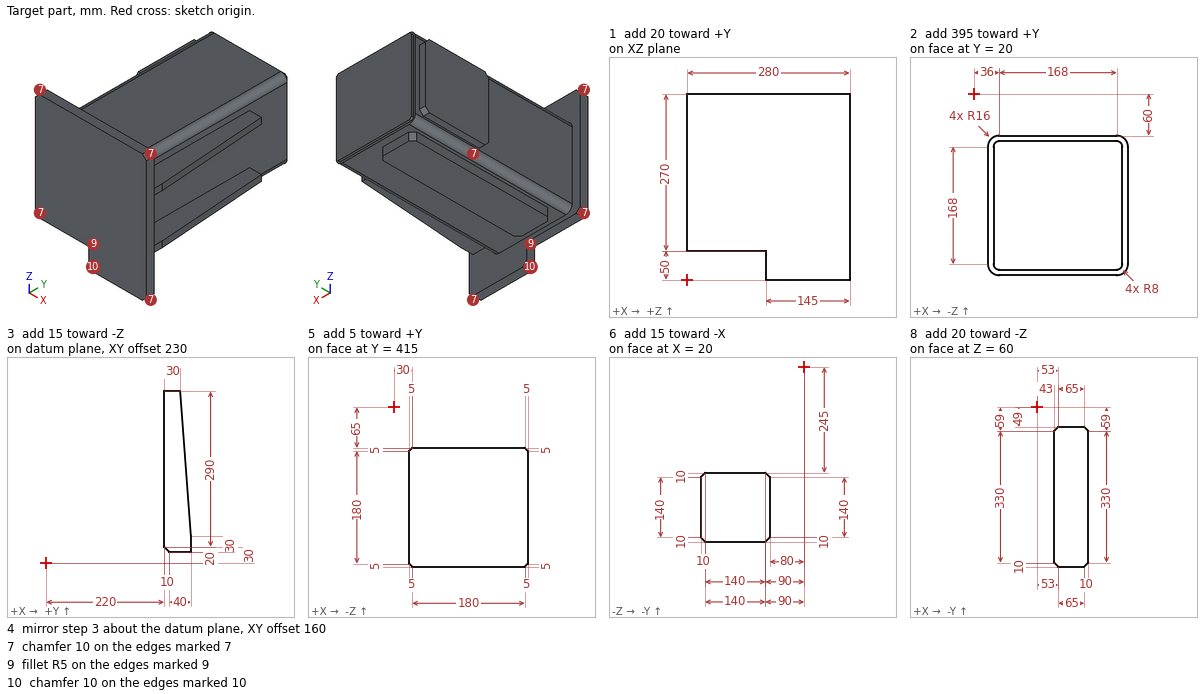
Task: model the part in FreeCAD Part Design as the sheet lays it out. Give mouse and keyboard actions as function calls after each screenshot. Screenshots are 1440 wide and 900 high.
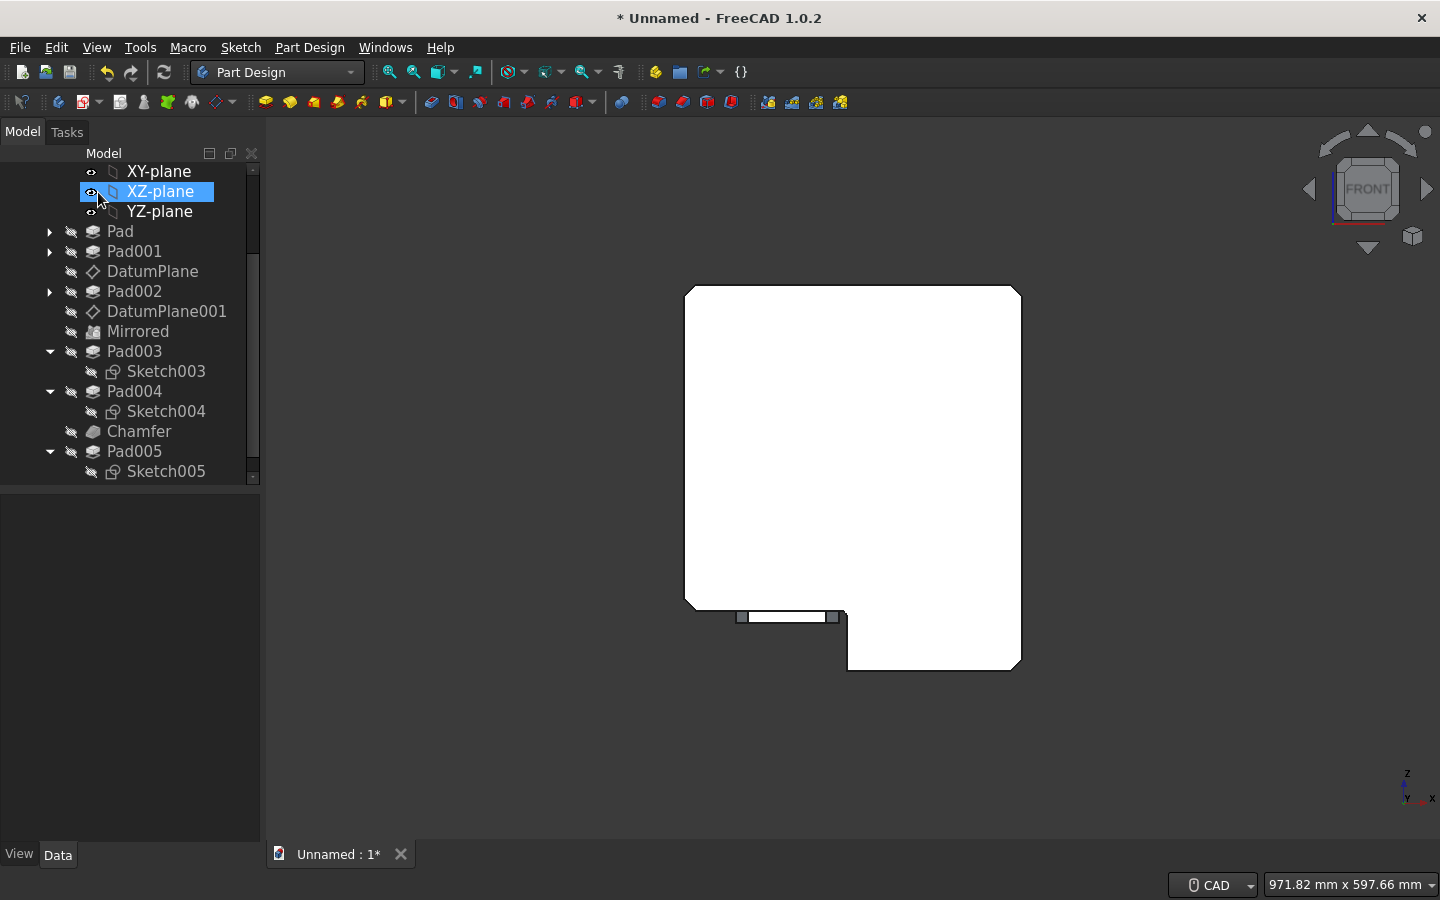
key(3)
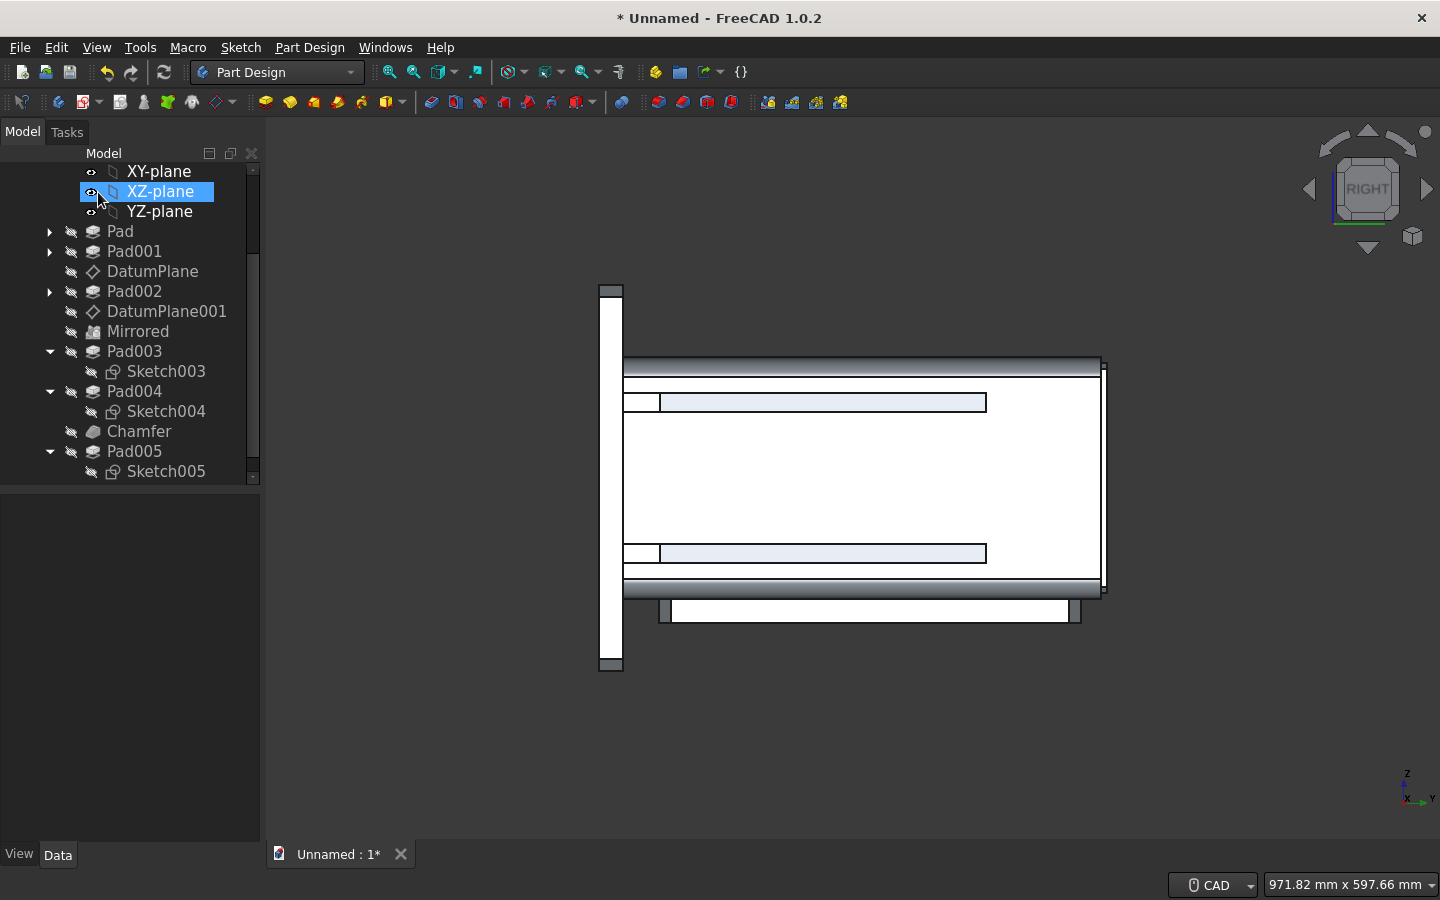
key(5)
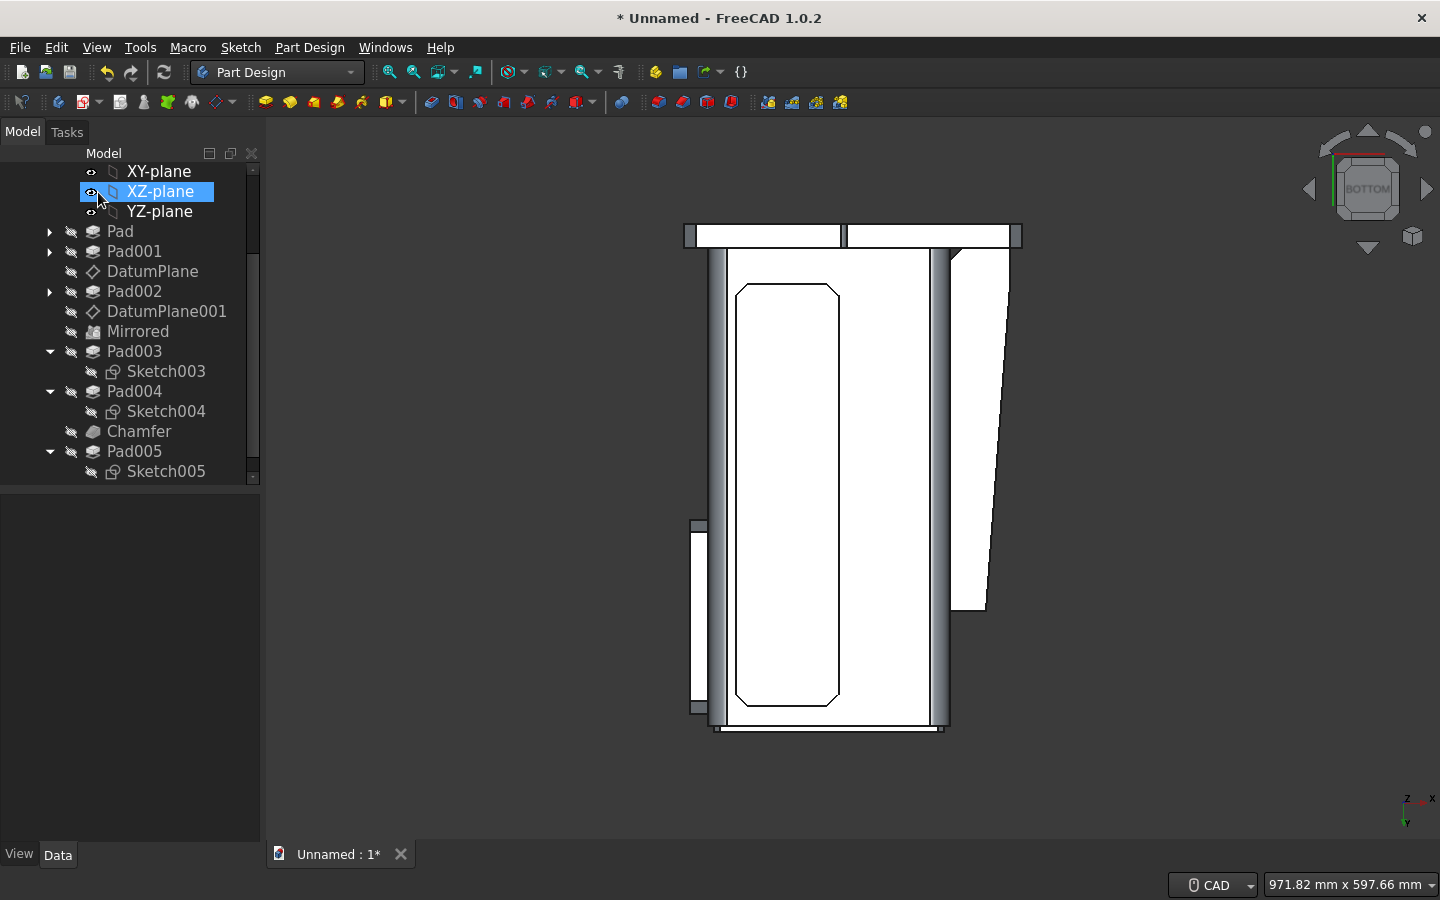
click(847, 235)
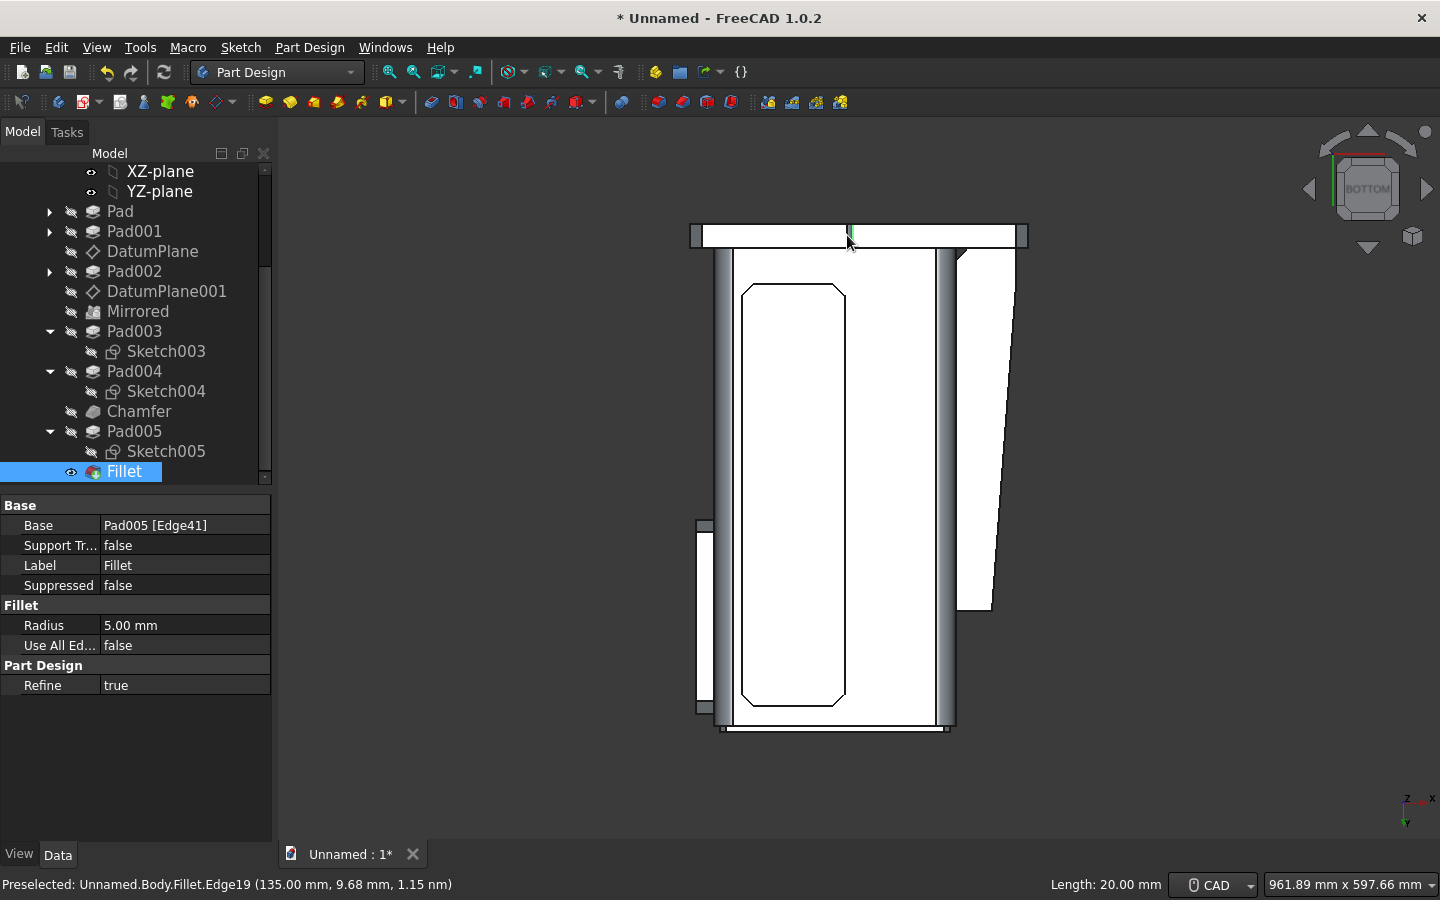
click(684, 102)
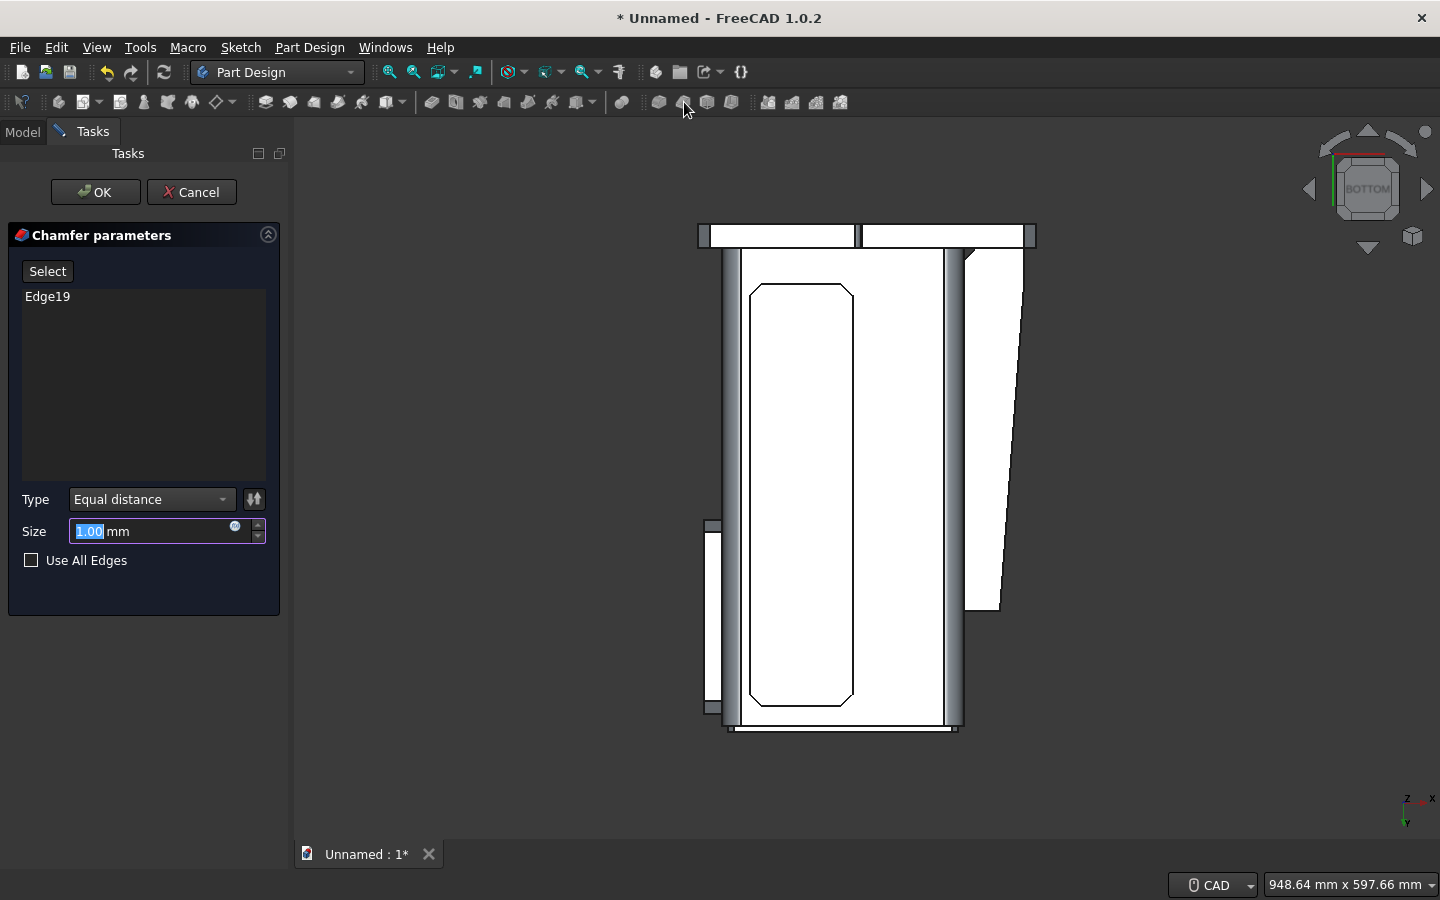
text(10)
key(Tab)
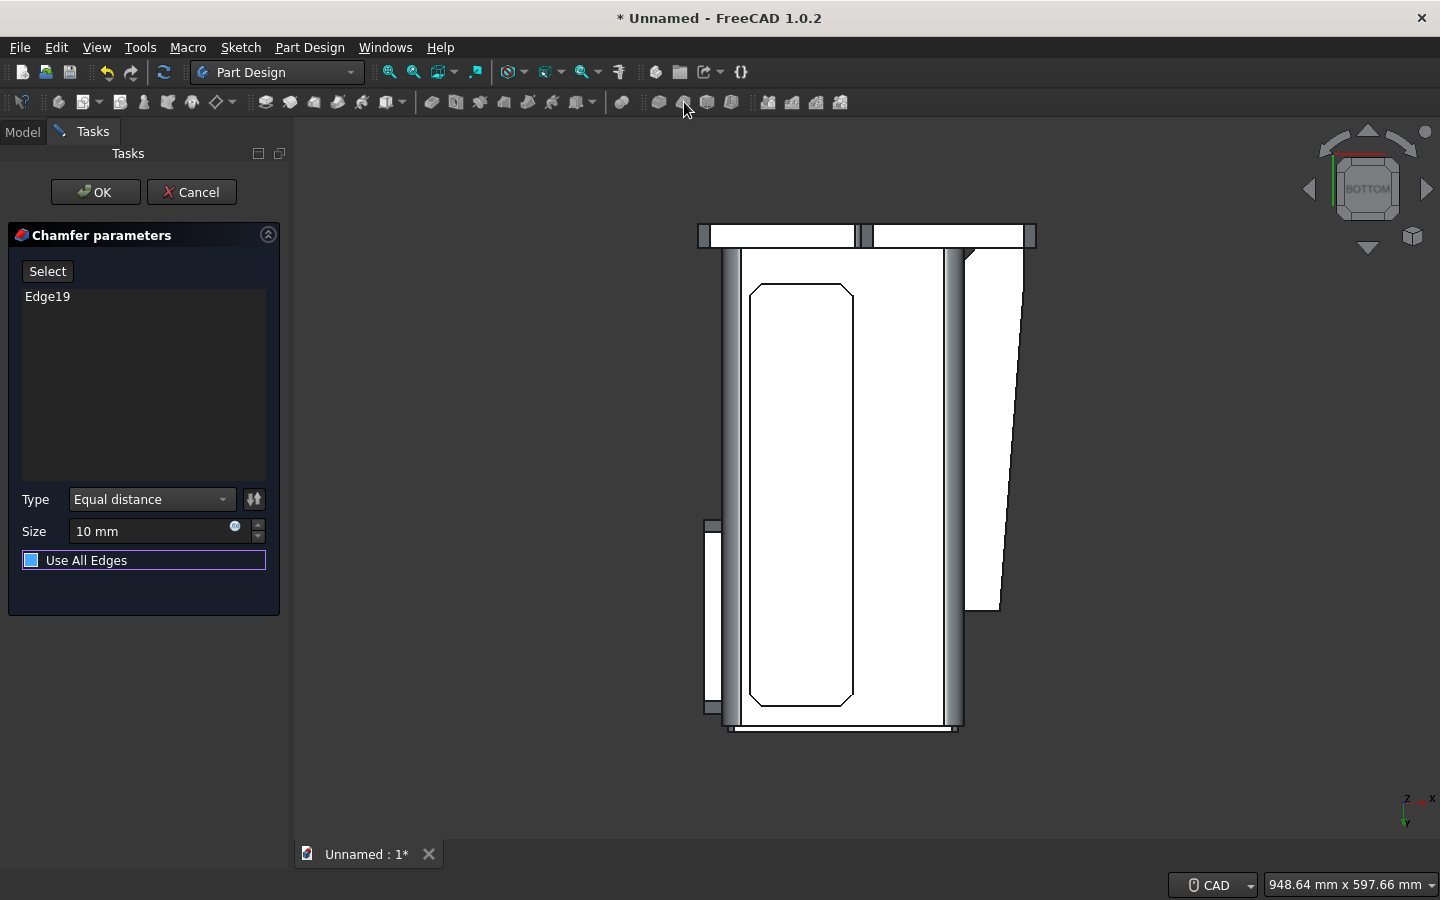
click(96, 192)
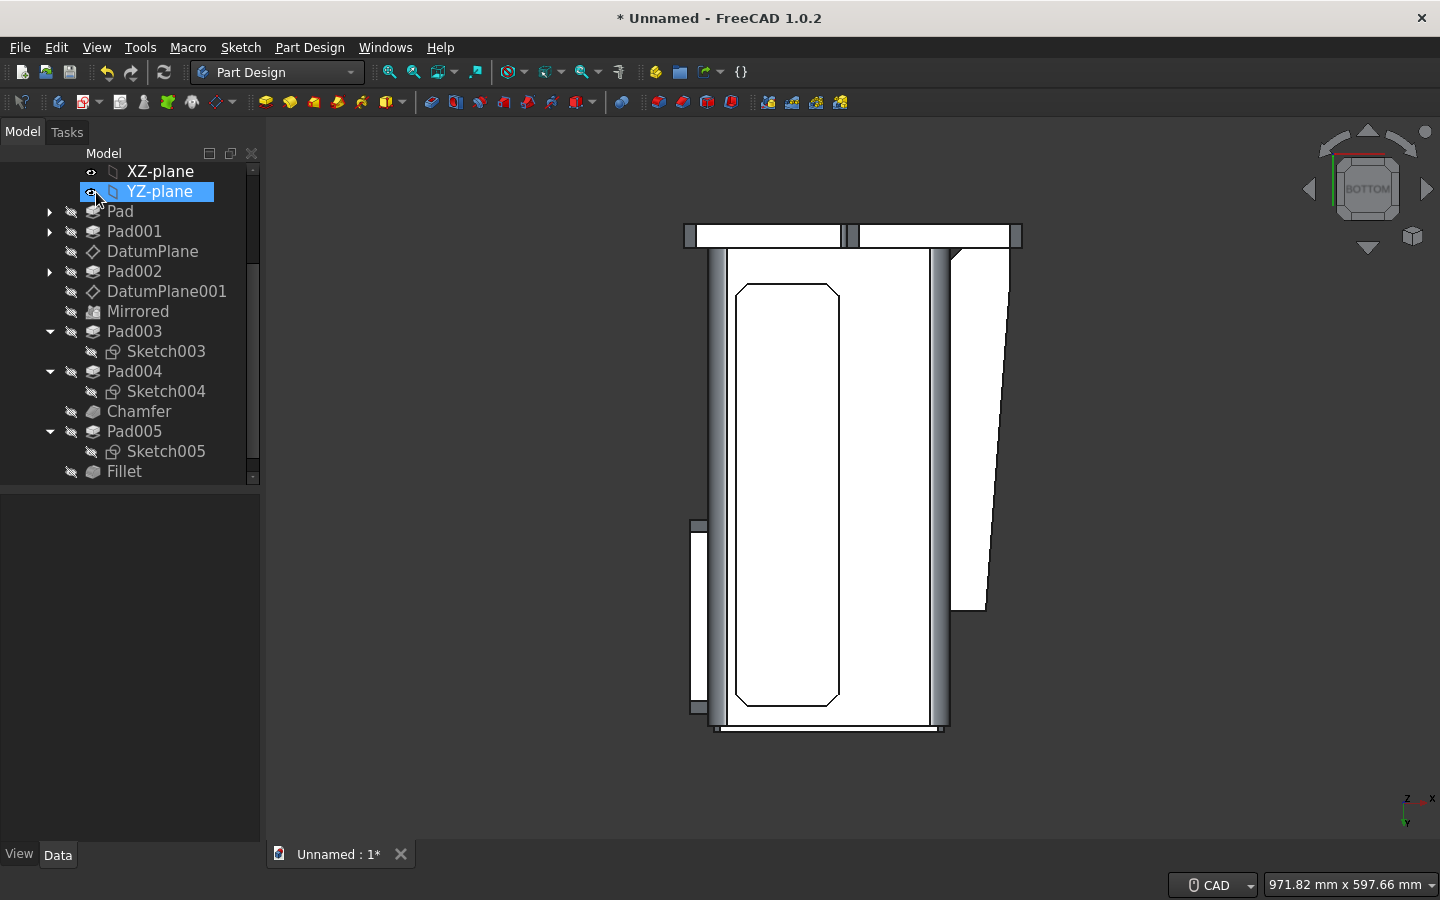
key(0)